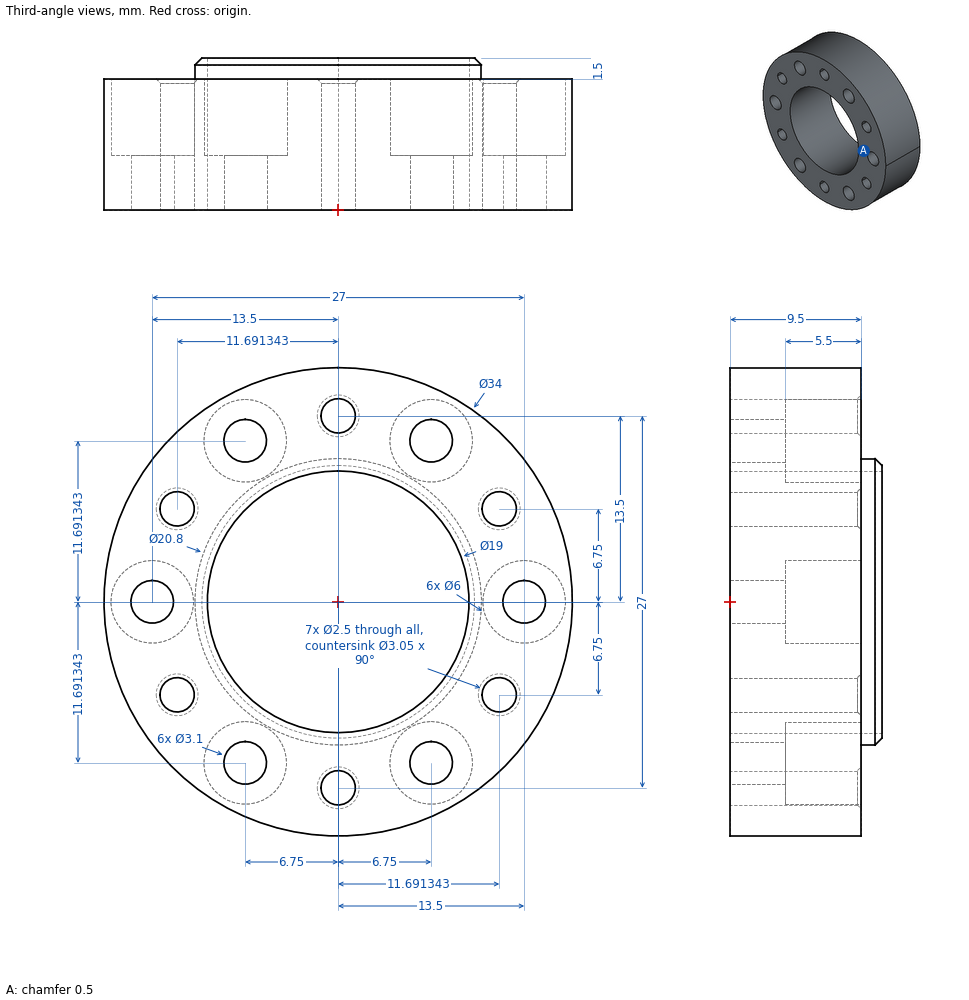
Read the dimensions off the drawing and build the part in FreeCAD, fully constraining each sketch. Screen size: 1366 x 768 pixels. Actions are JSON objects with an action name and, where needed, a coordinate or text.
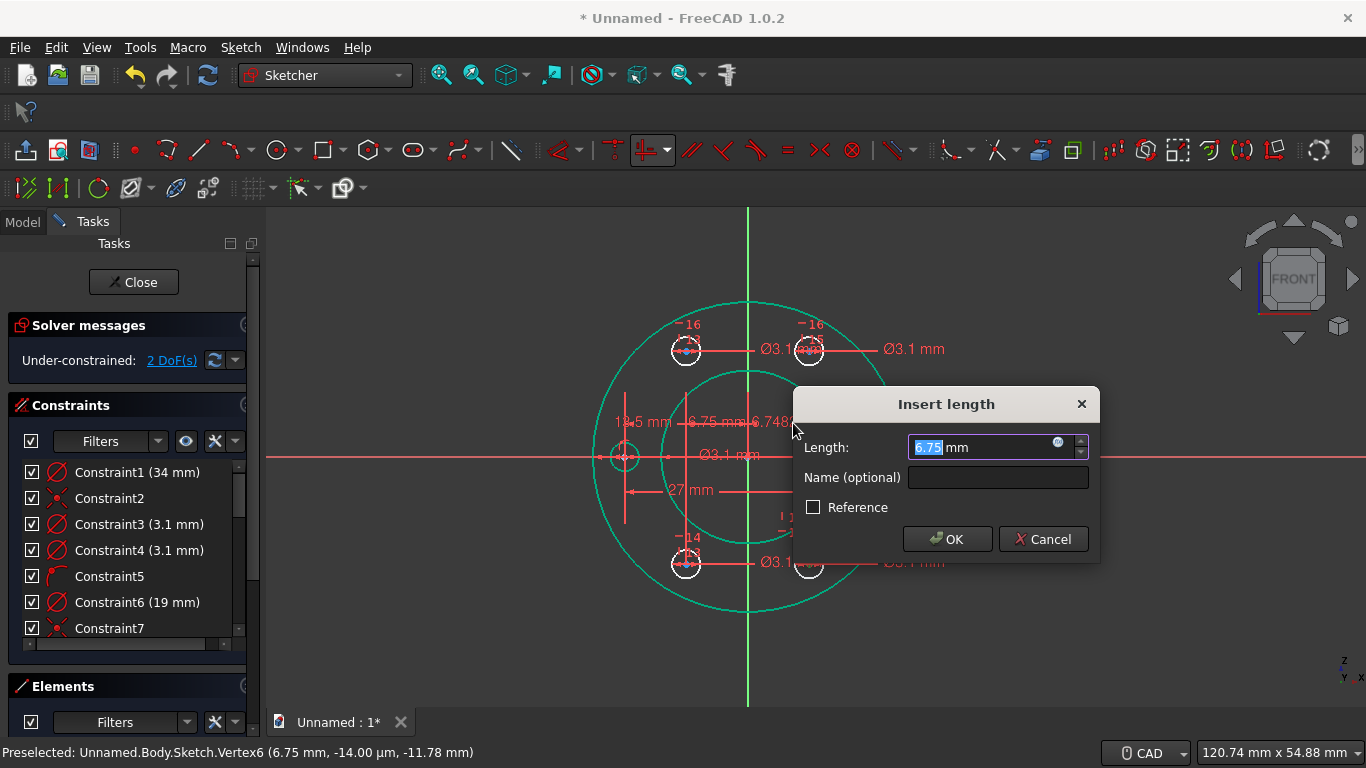
{"action": "type", "text": "6.75"}
{"action": "key", "text": "Return"}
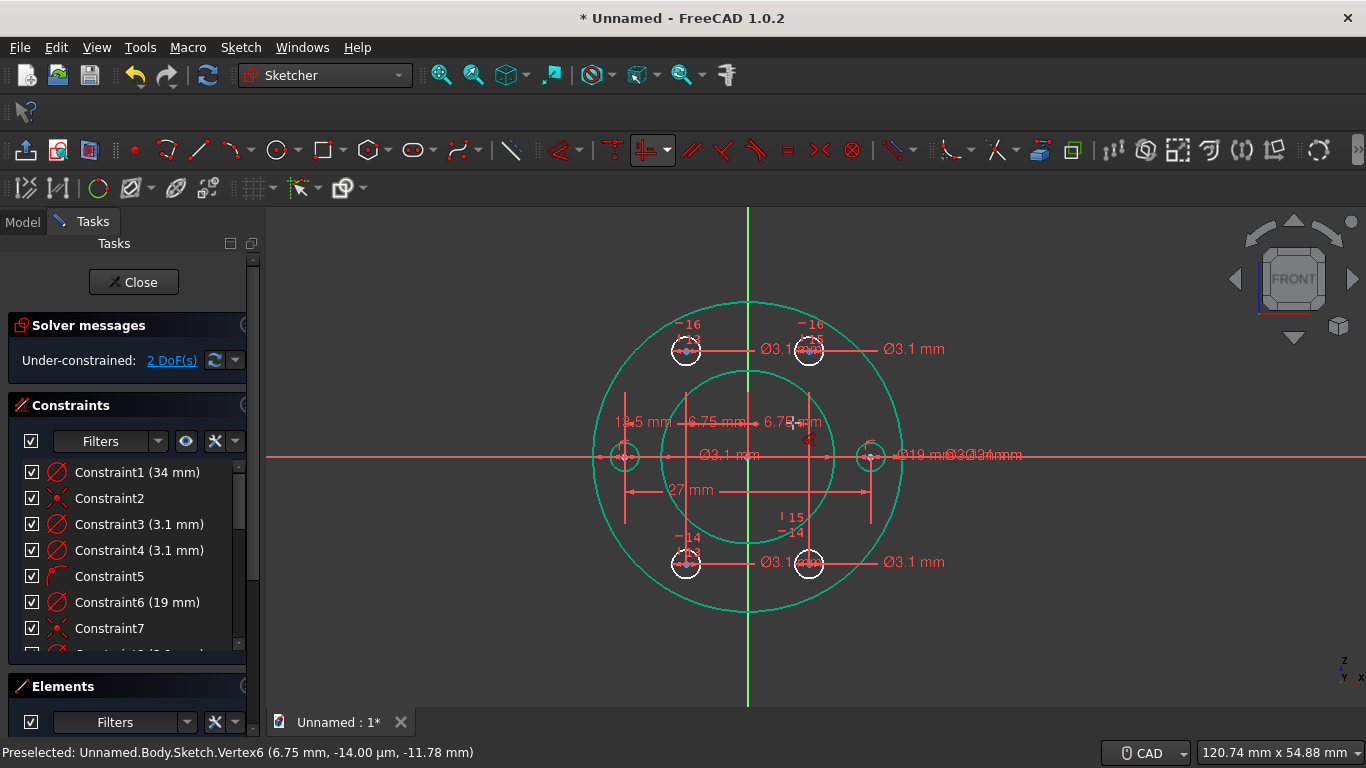
{"action": "left_click", "coordinate": [686, 564]}
{"action": "left_click", "coordinate": [652, 535]}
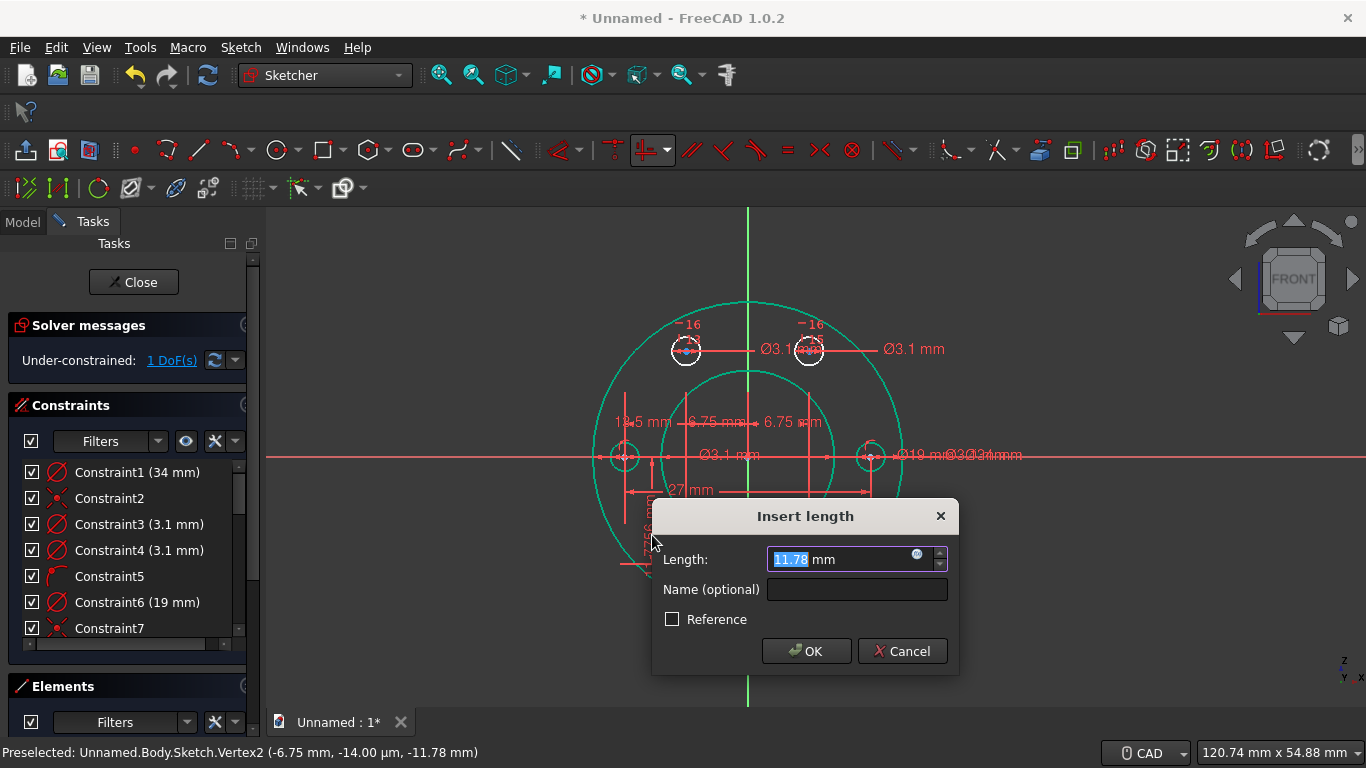
{"action": "type", "text": "11.691343"}
{"action": "key", "text": "Return"}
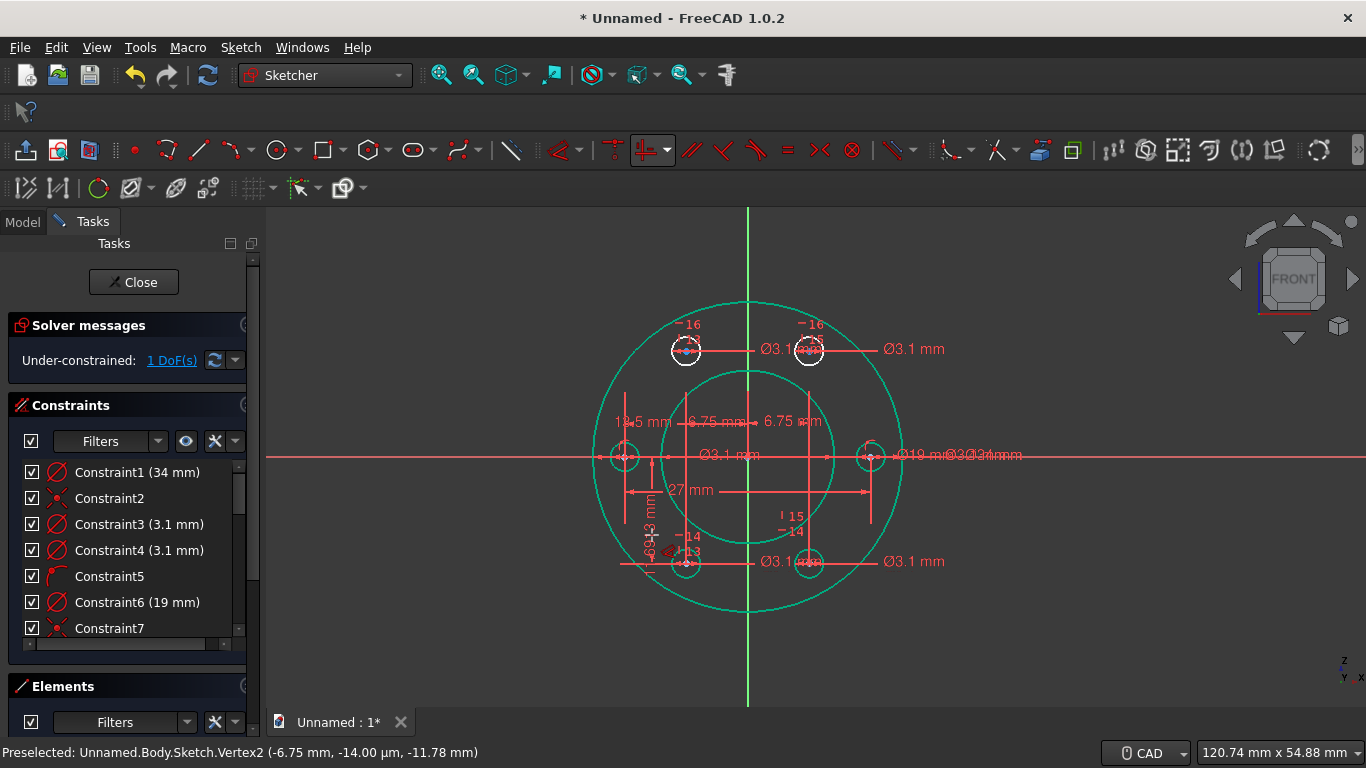
{"action": "left_click", "coordinate": [686, 351]}
{"action": "left_click", "coordinate": [652, 380]}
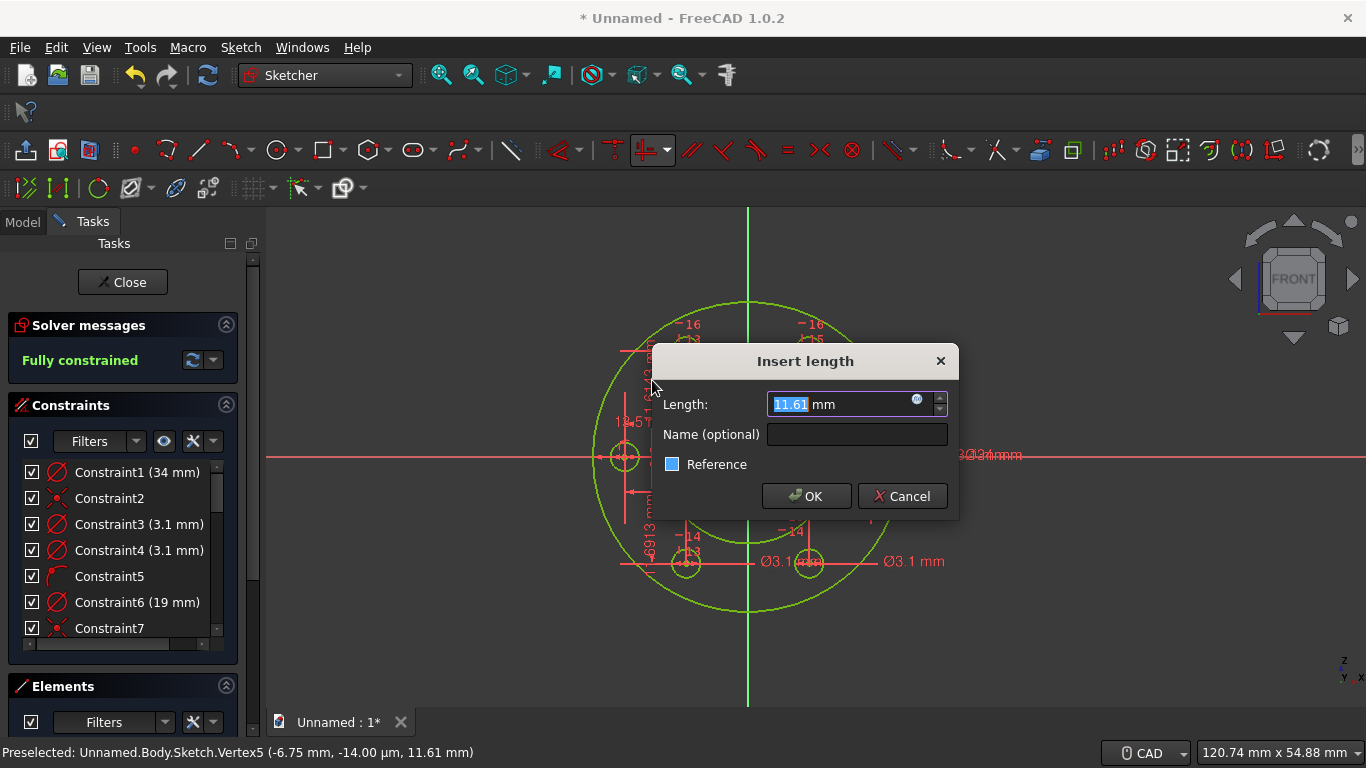
{"action": "type", "text": "11.691343"}
{"action": "key", "text": "Return"}
{"action": "key", "text": "Escape"}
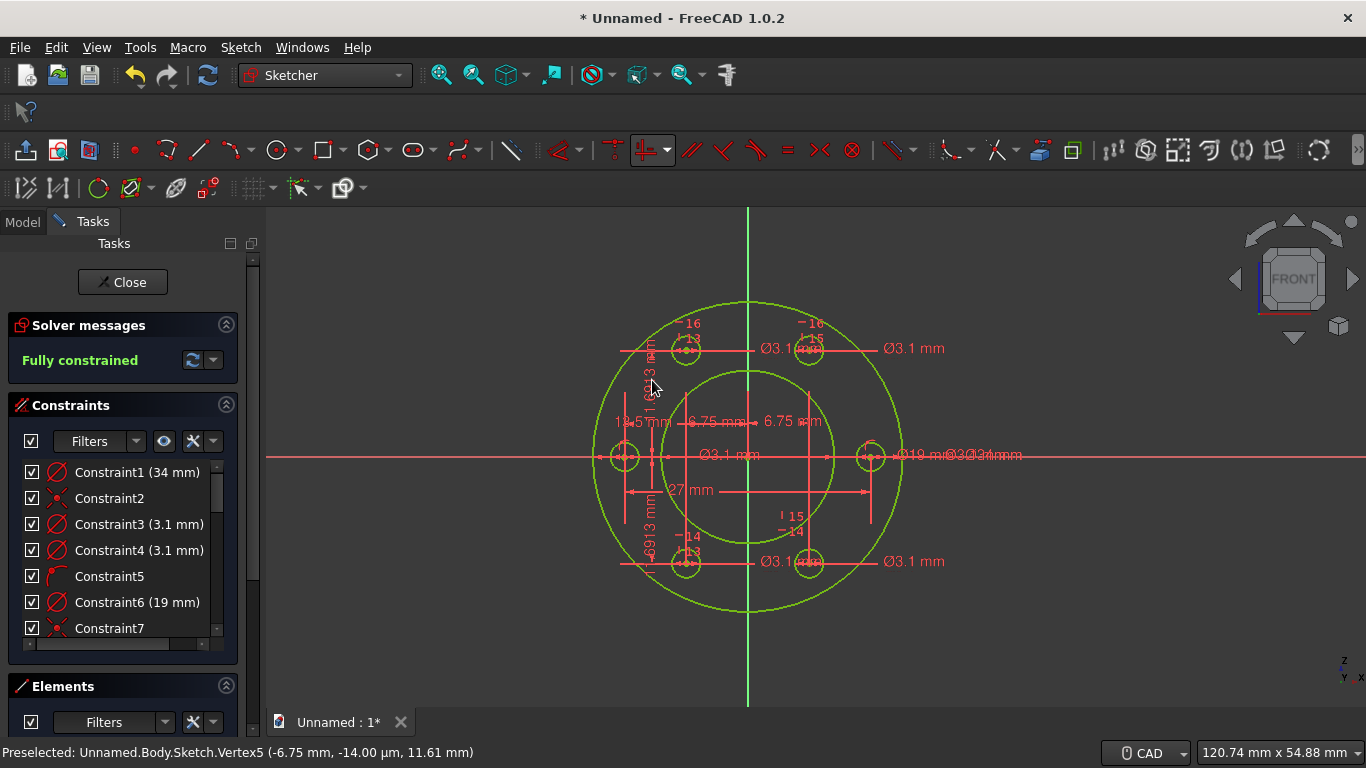
{"action": "left_click", "coordinate": [123, 282]}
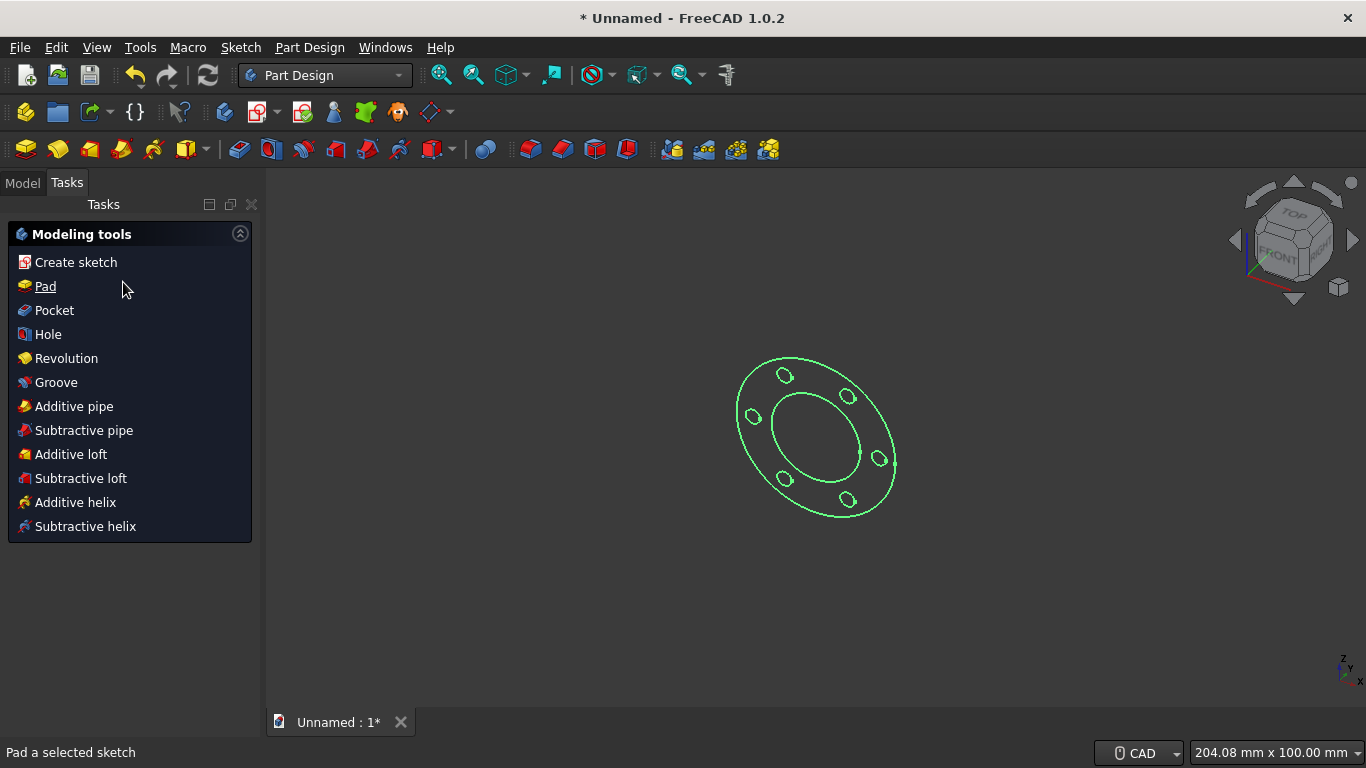
{"action": "left_click", "coordinate": [26, 150]}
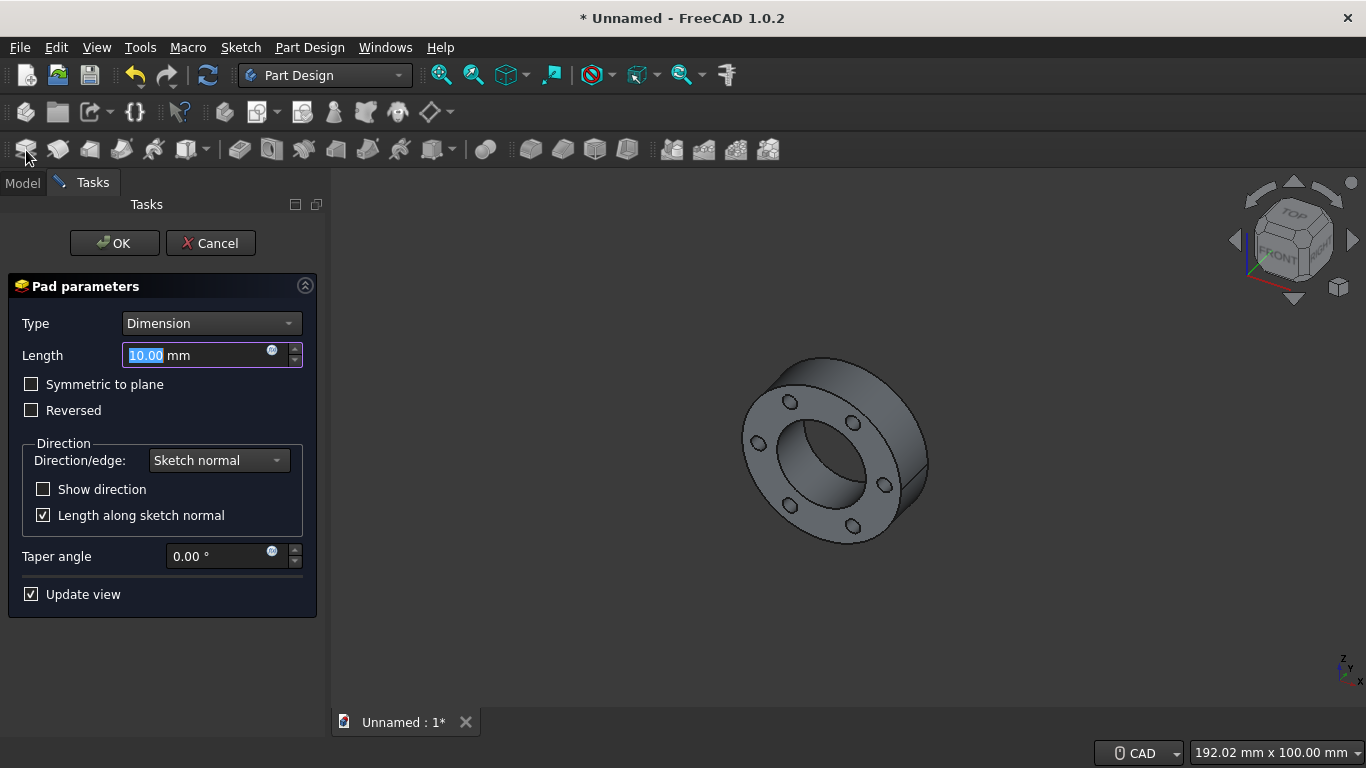
{"action": "type", "text": "9.5"}
{"action": "key", "text": "Tab"}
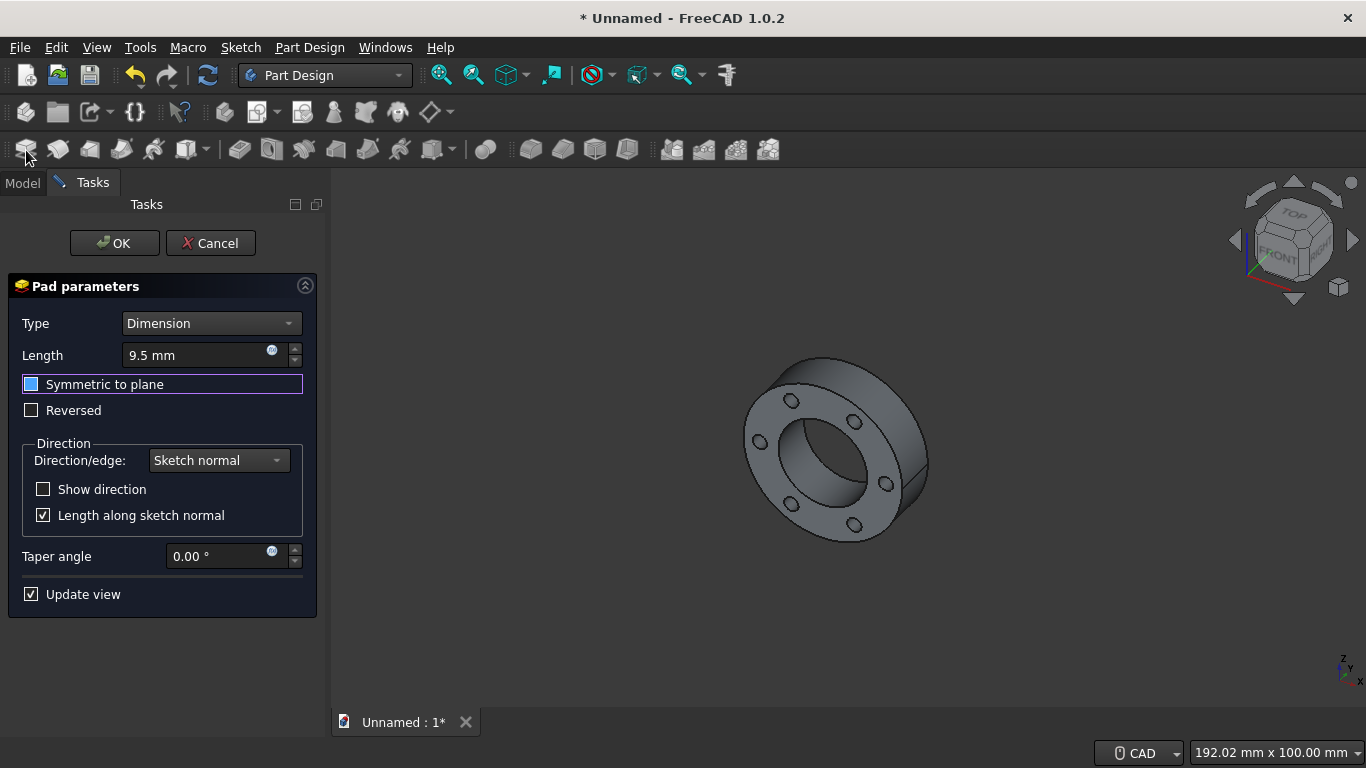
{"action": "left_click", "coordinate": [30, 410]}